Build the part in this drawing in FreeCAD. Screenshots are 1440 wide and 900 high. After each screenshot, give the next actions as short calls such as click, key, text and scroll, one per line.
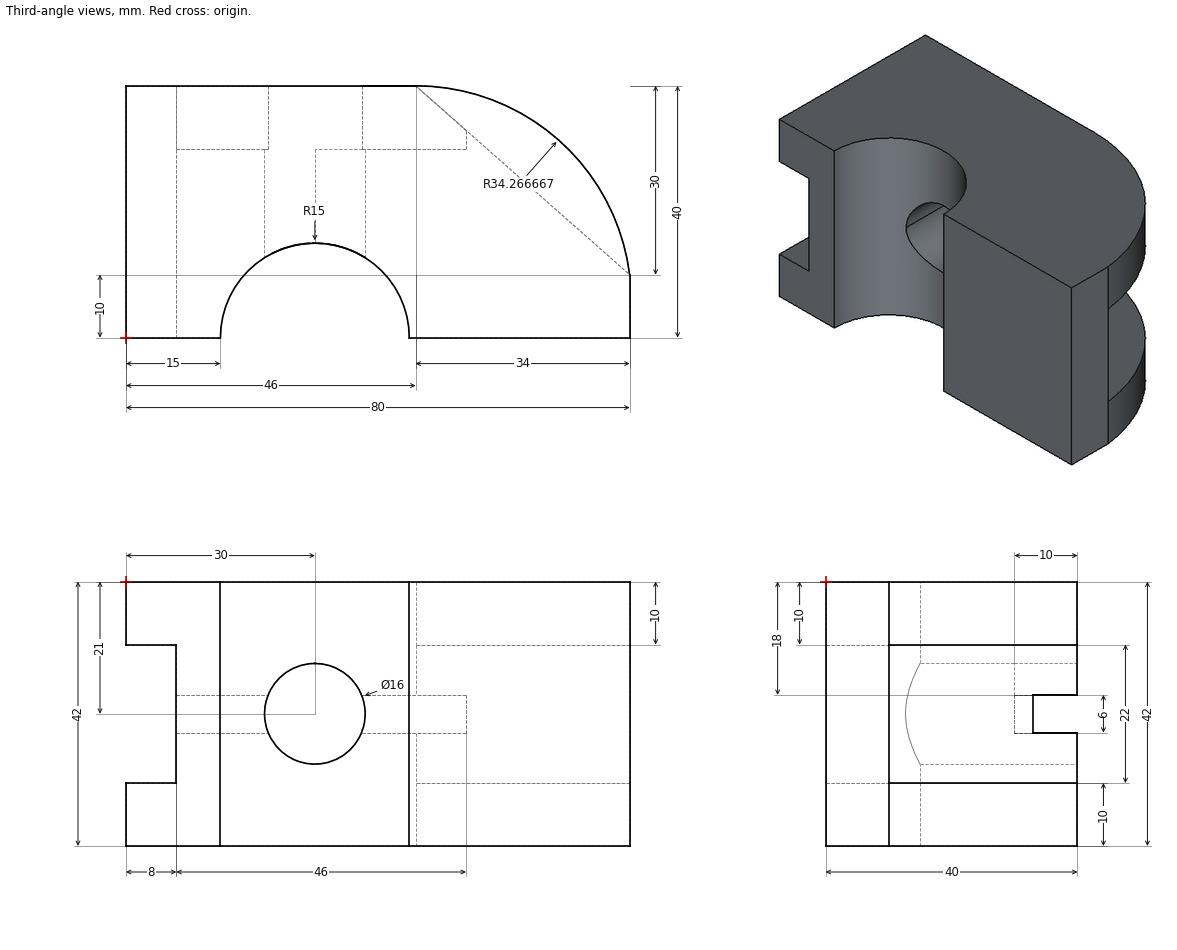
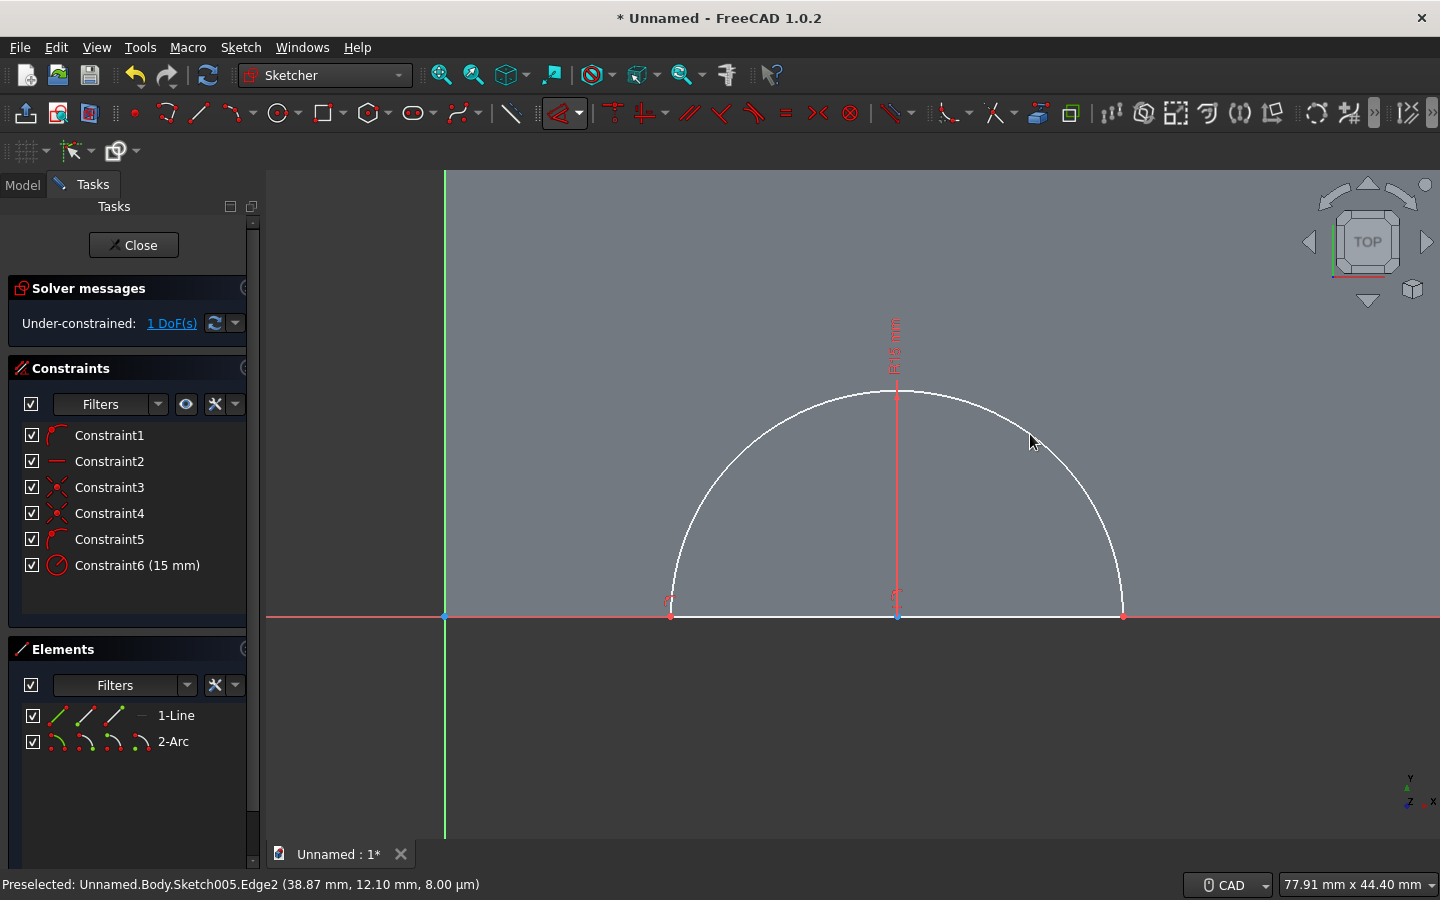
click(671, 617)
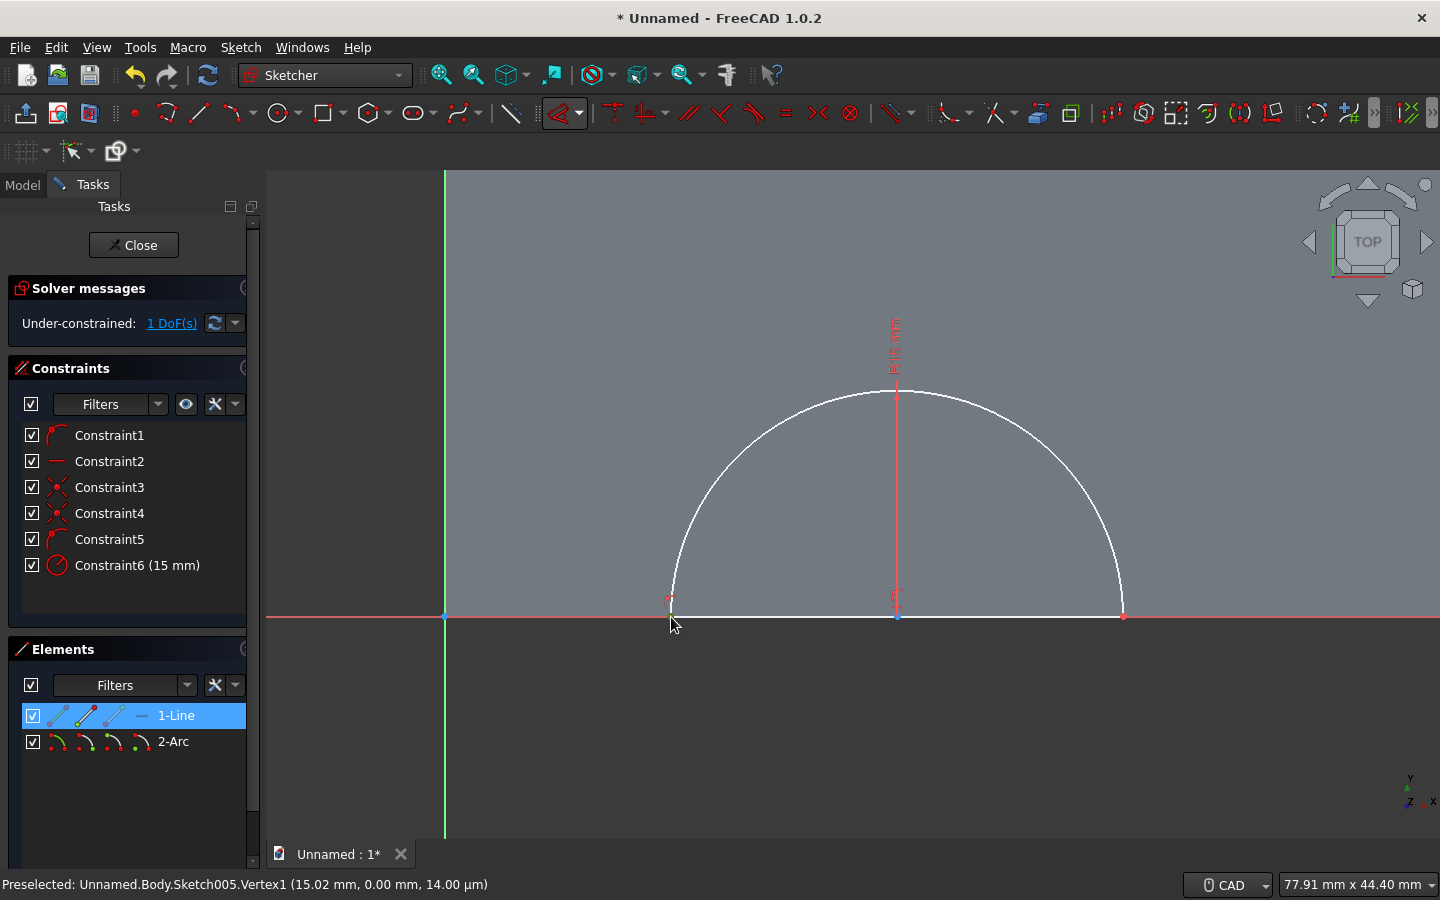
key(l)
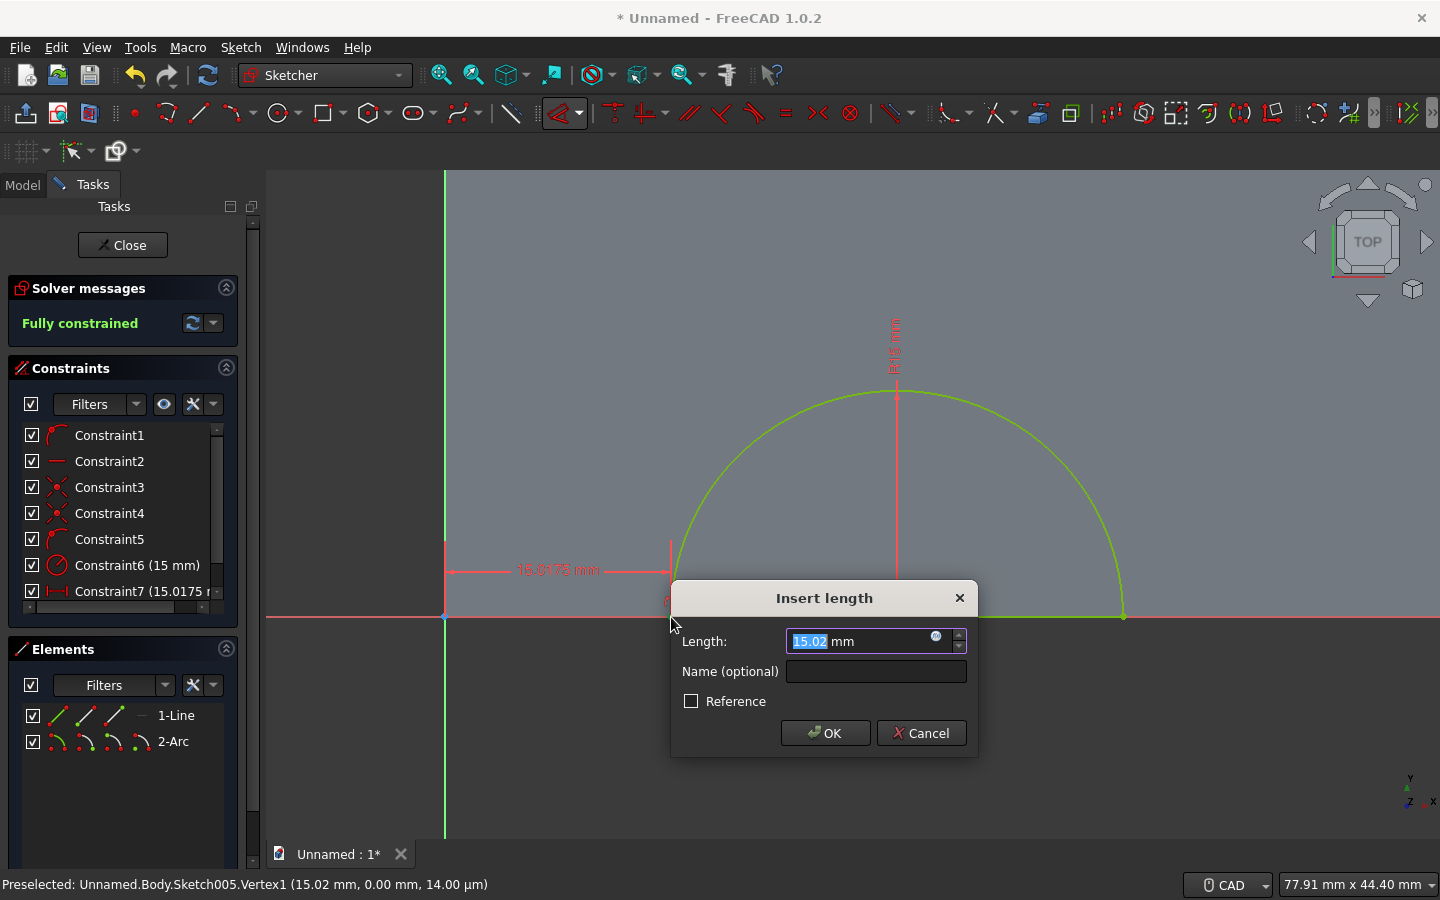
text(15)
key(Return)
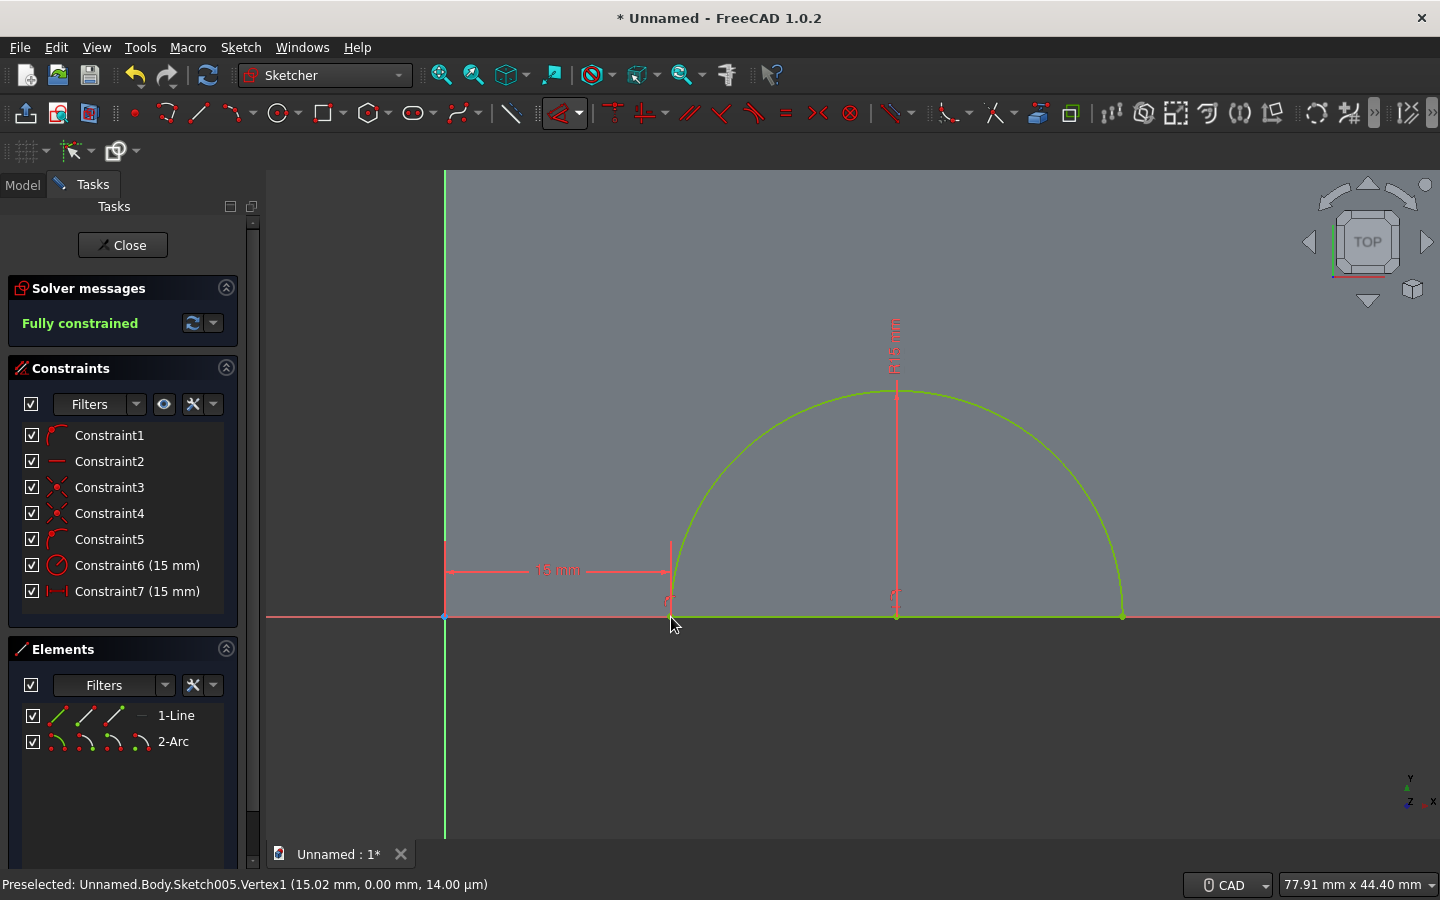
click(123, 245)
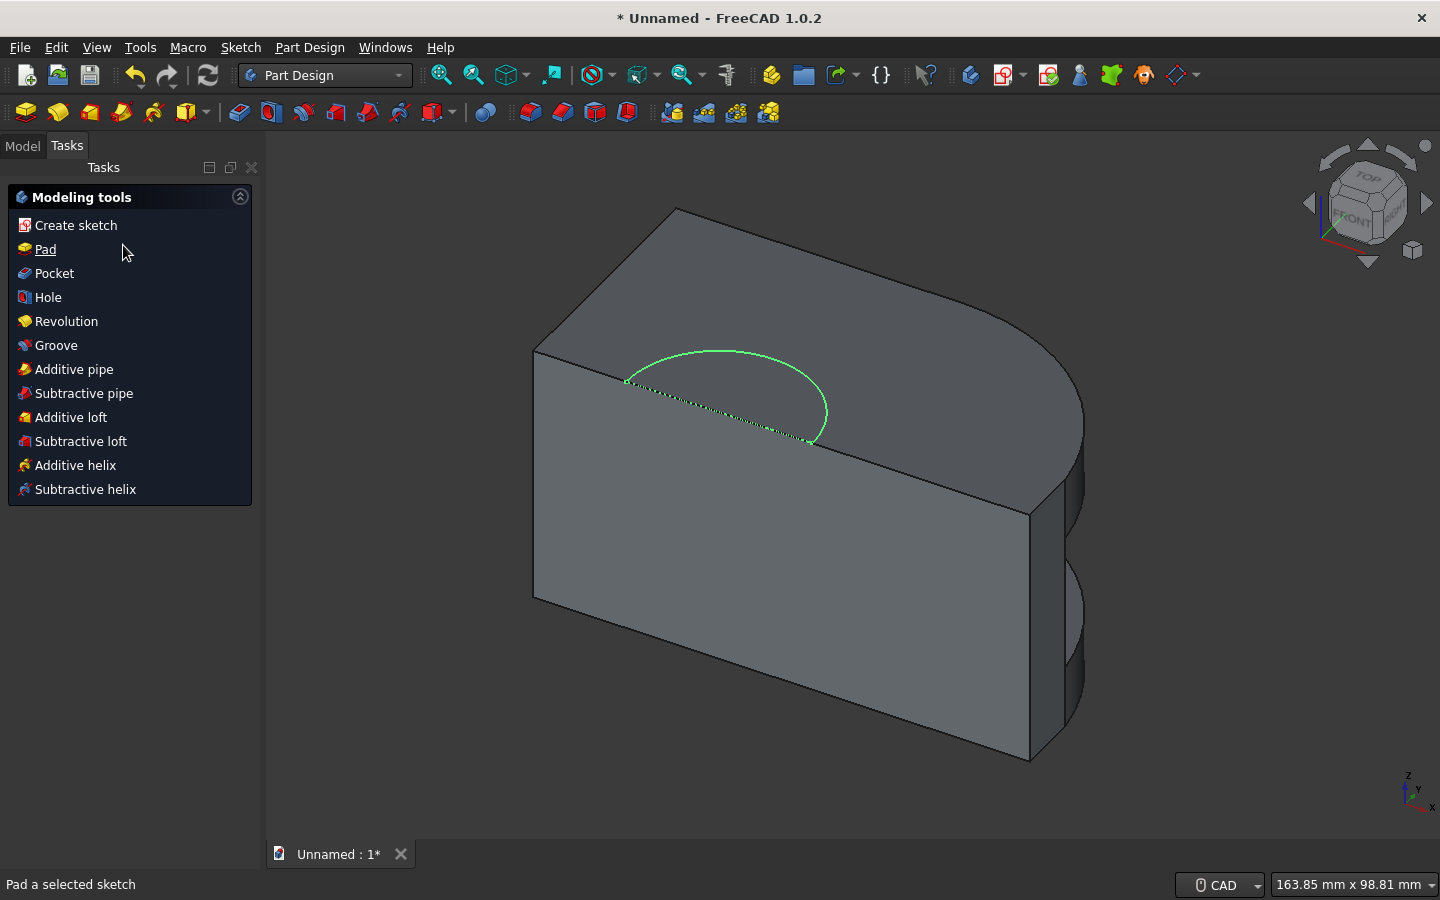
click(240, 112)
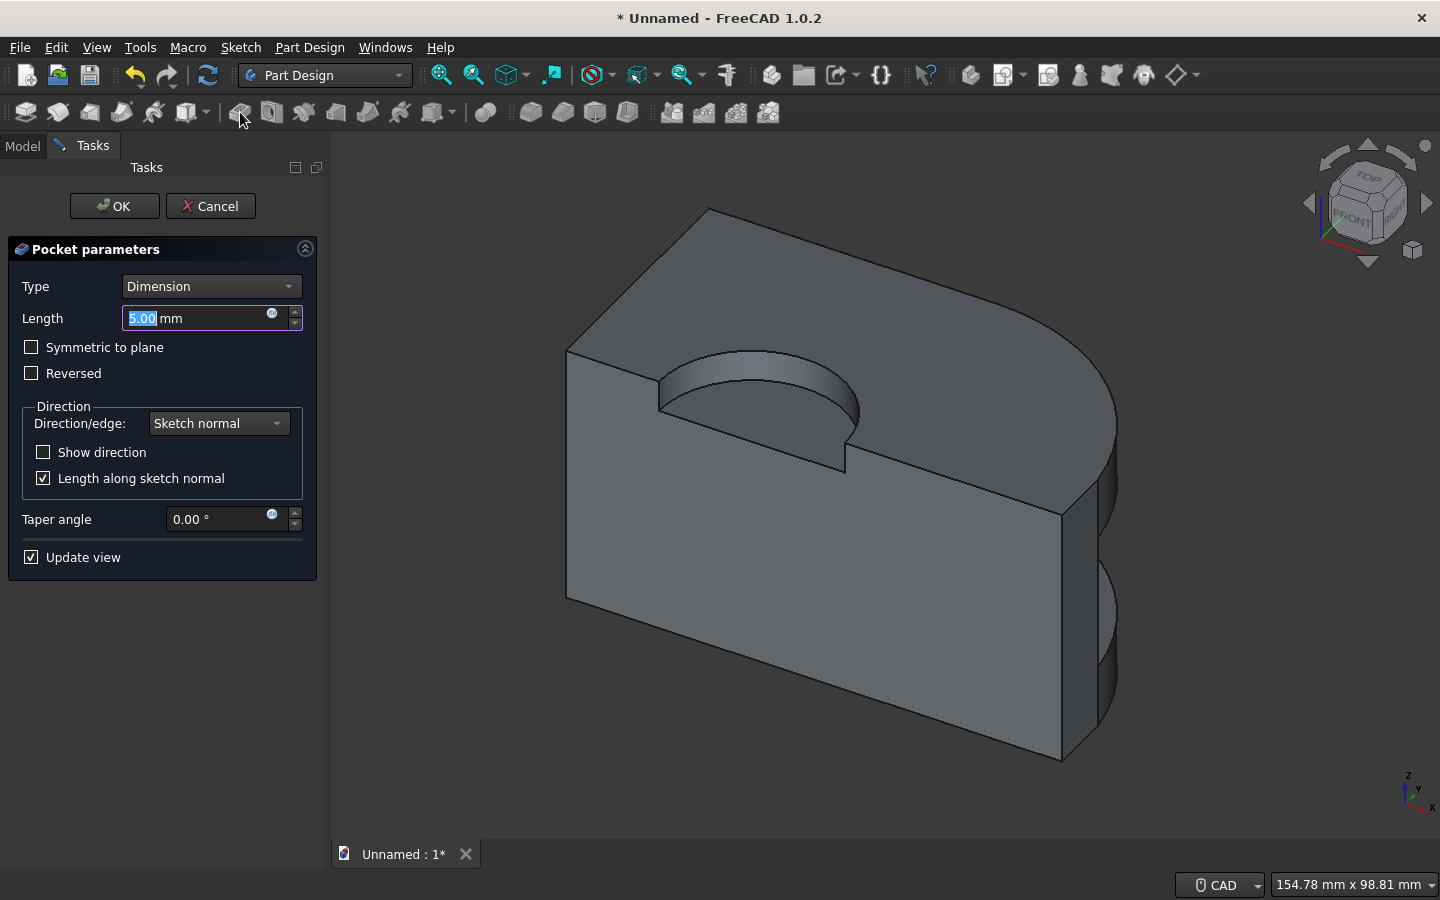
text(42)
key(Tab)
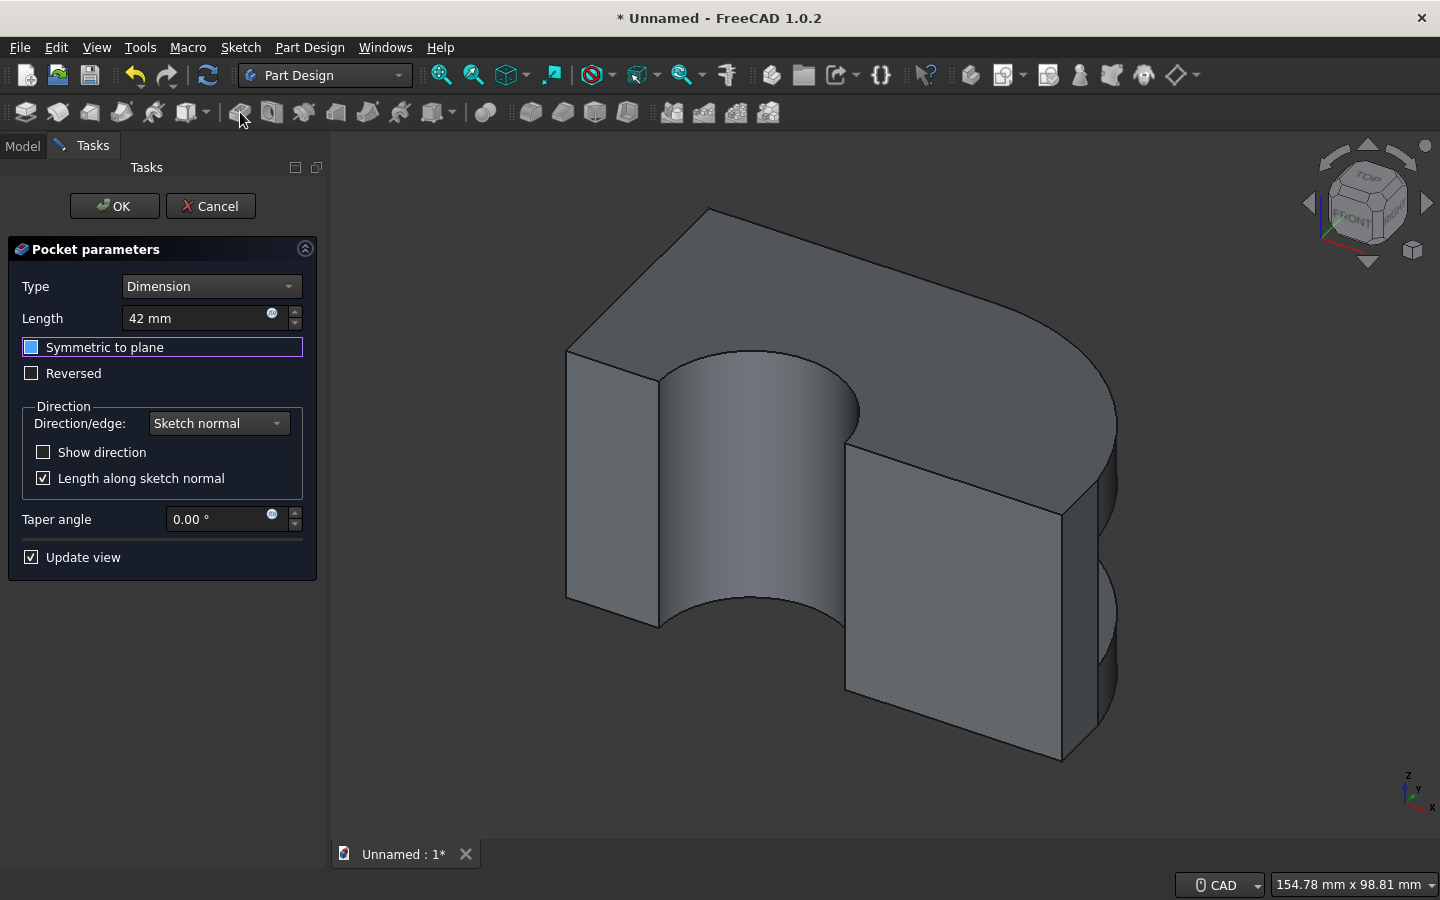
click(115, 206)